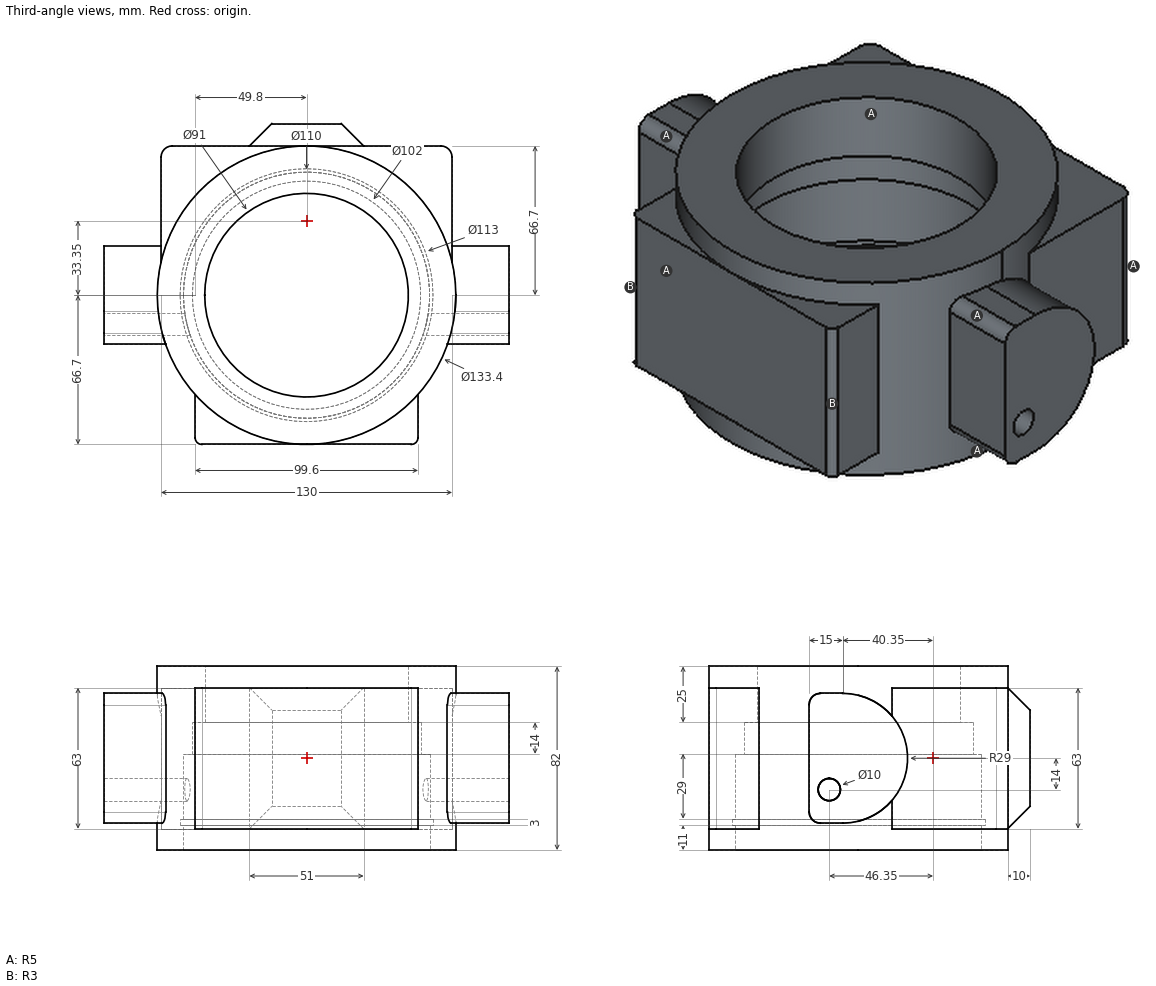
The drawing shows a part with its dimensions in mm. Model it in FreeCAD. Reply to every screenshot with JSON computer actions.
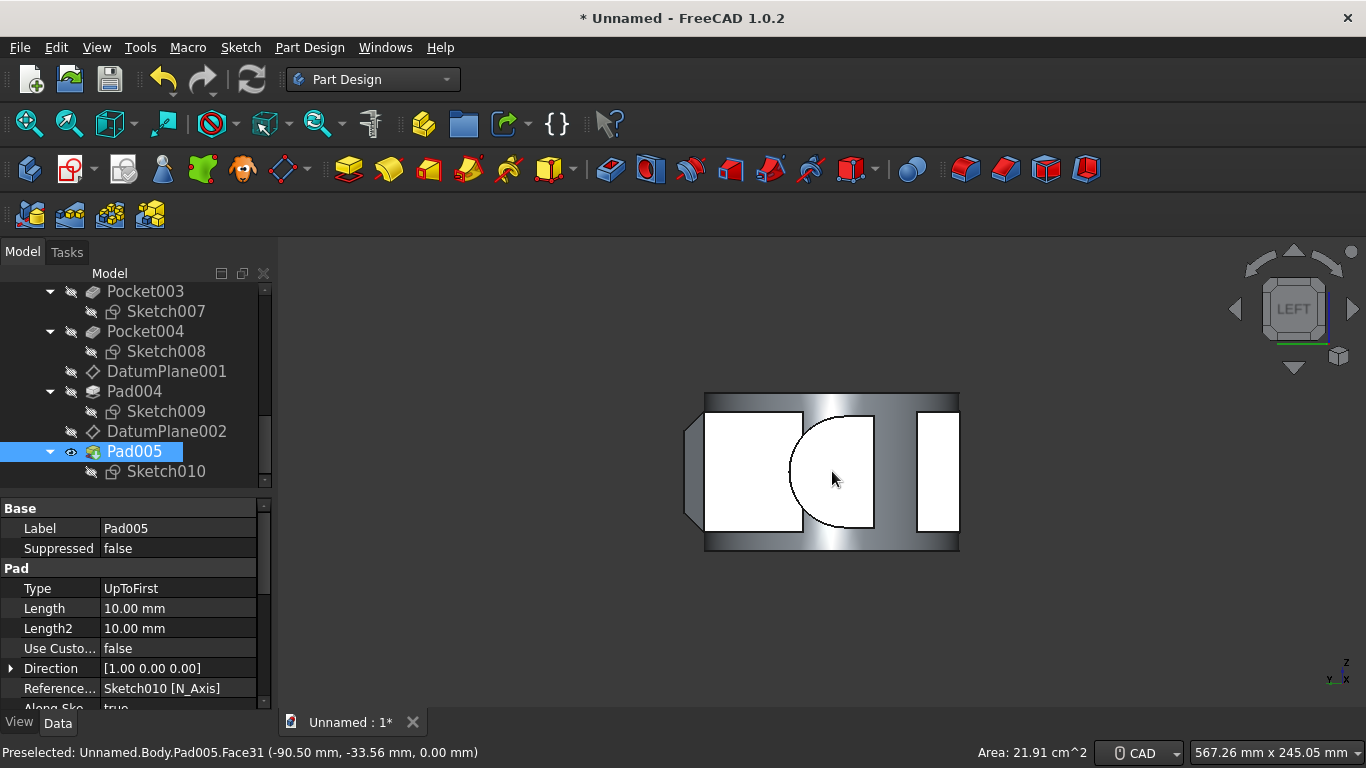
{"action": "left_click", "coordinate": [70, 170]}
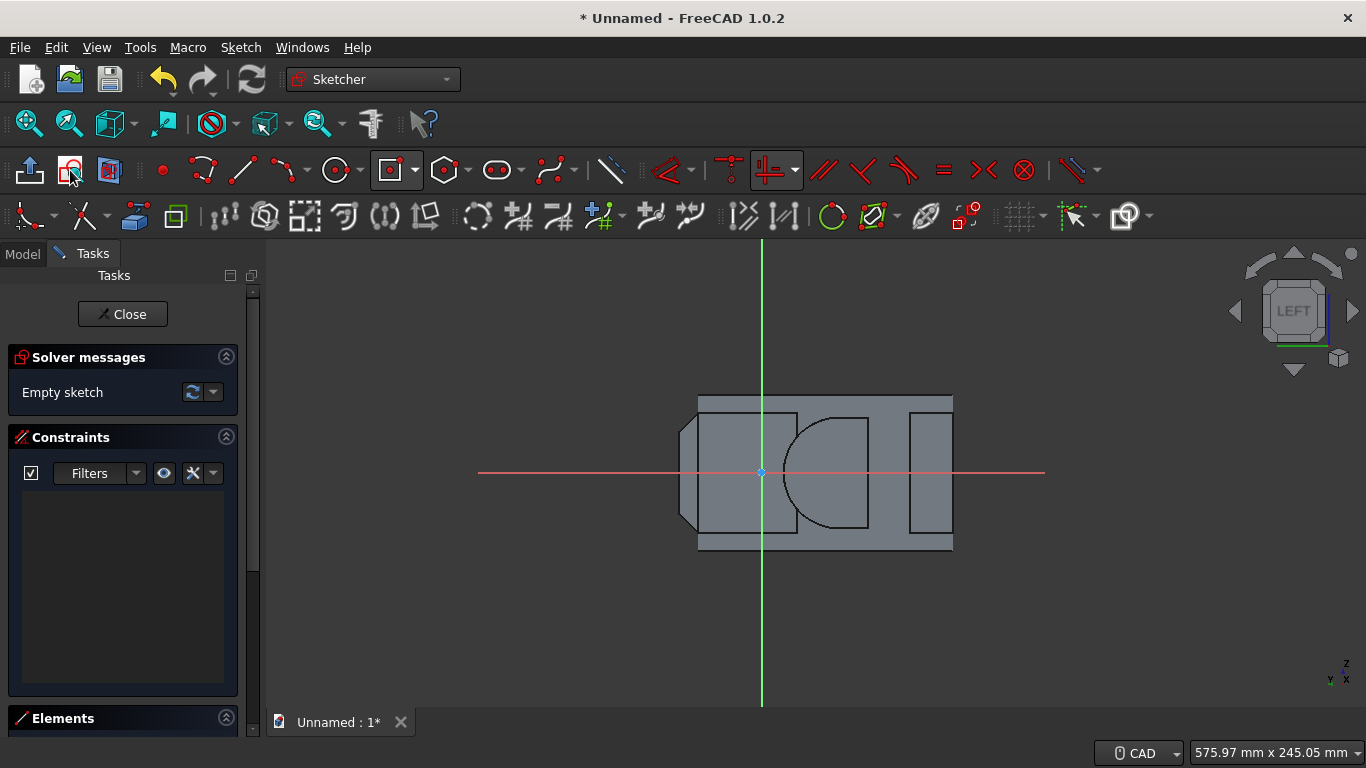
{"action": "scroll", "coordinate": [857, 501], "scroll_direction": "up", "scroll_amount": 14}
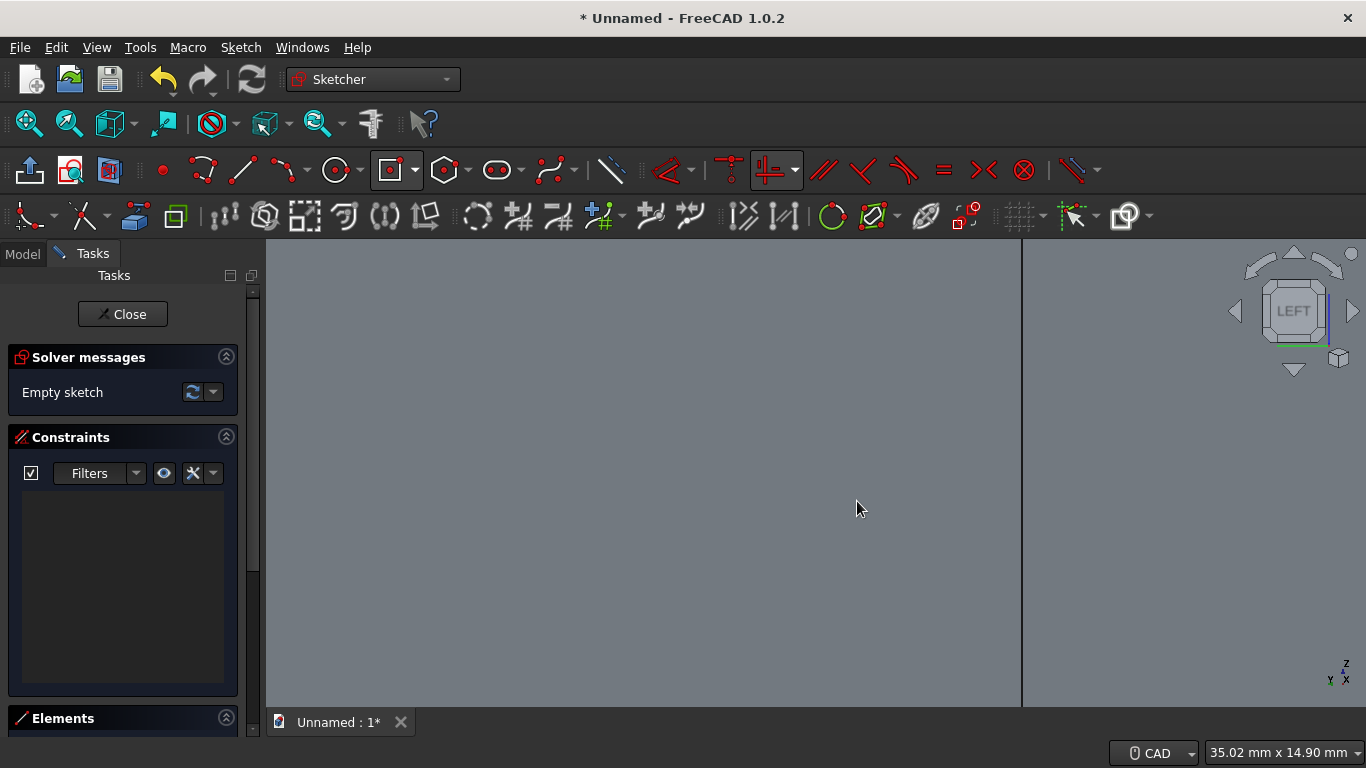
{"action": "left_click", "coordinate": [336, 170]}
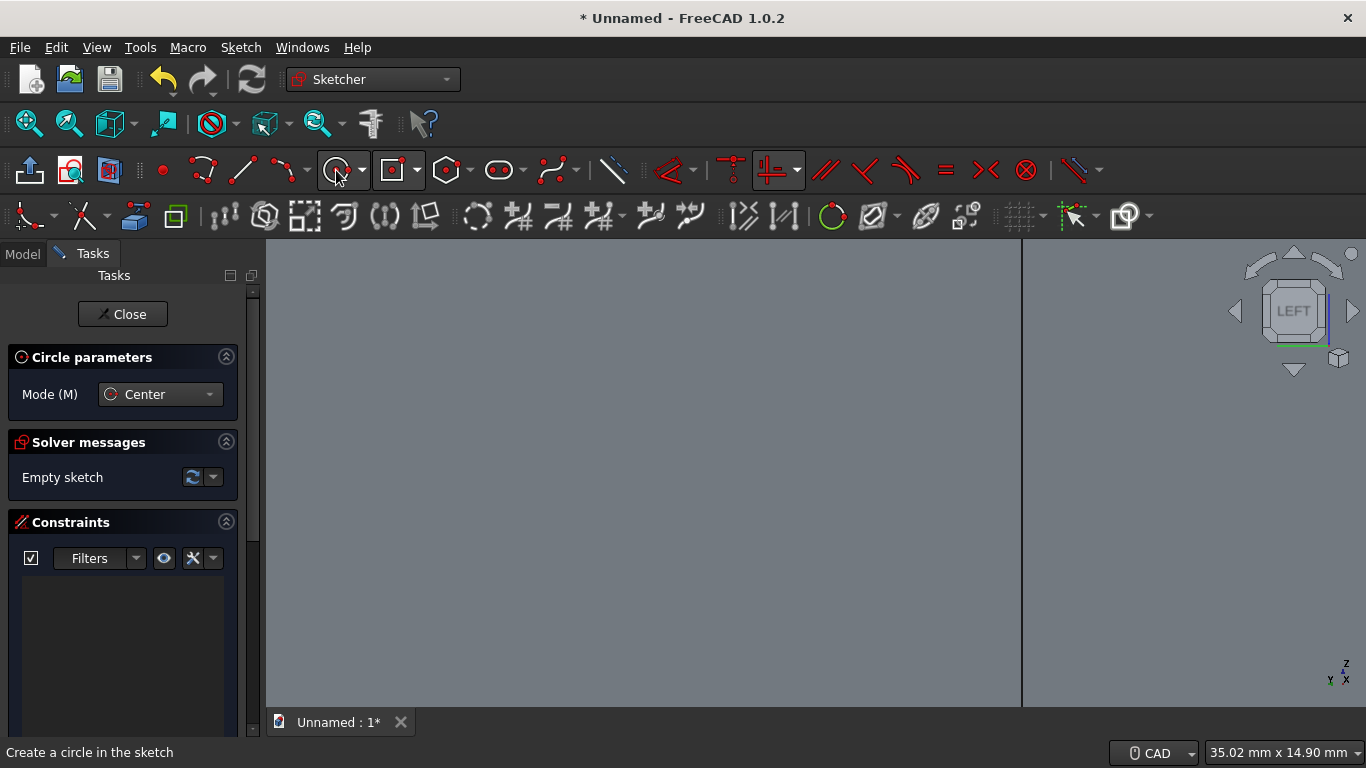
{"action": "left_click", "coordinate": [740, 472]}
{"action": "left_click", "coordinate": [851, 361]}
{"action": "key", "text": "Escape"}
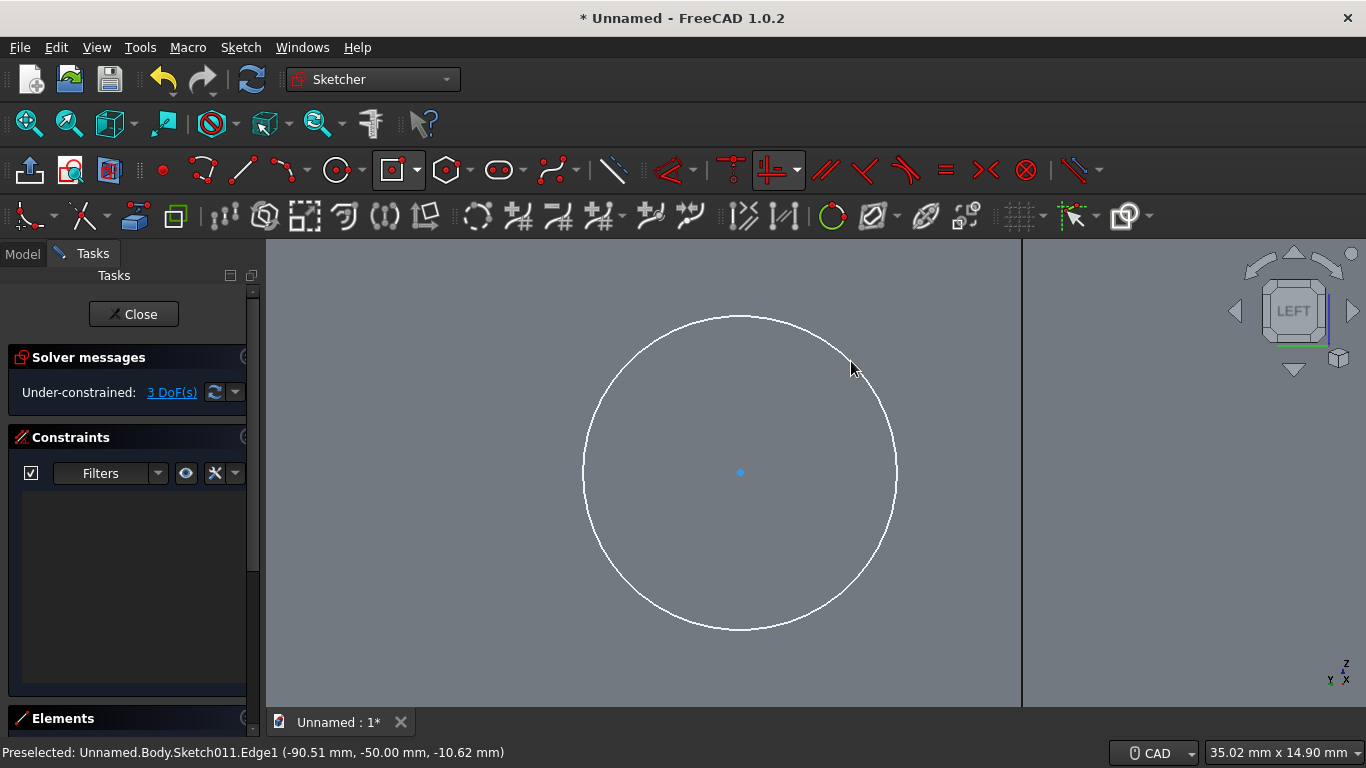
{"action": "key", "text": "d"}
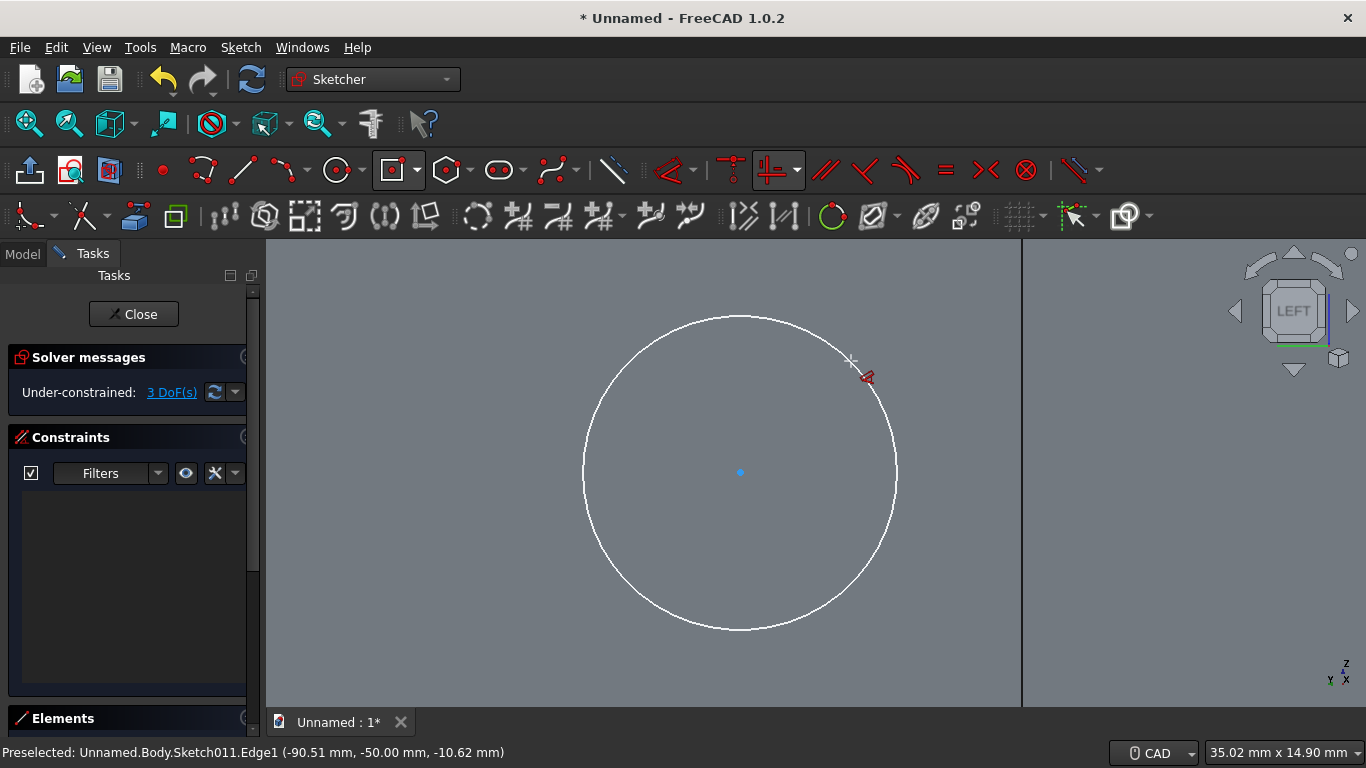
{"action": "left_click", "coordinate": [851, 362]}
{"action": "left_click", "coordinate": [874, 339]}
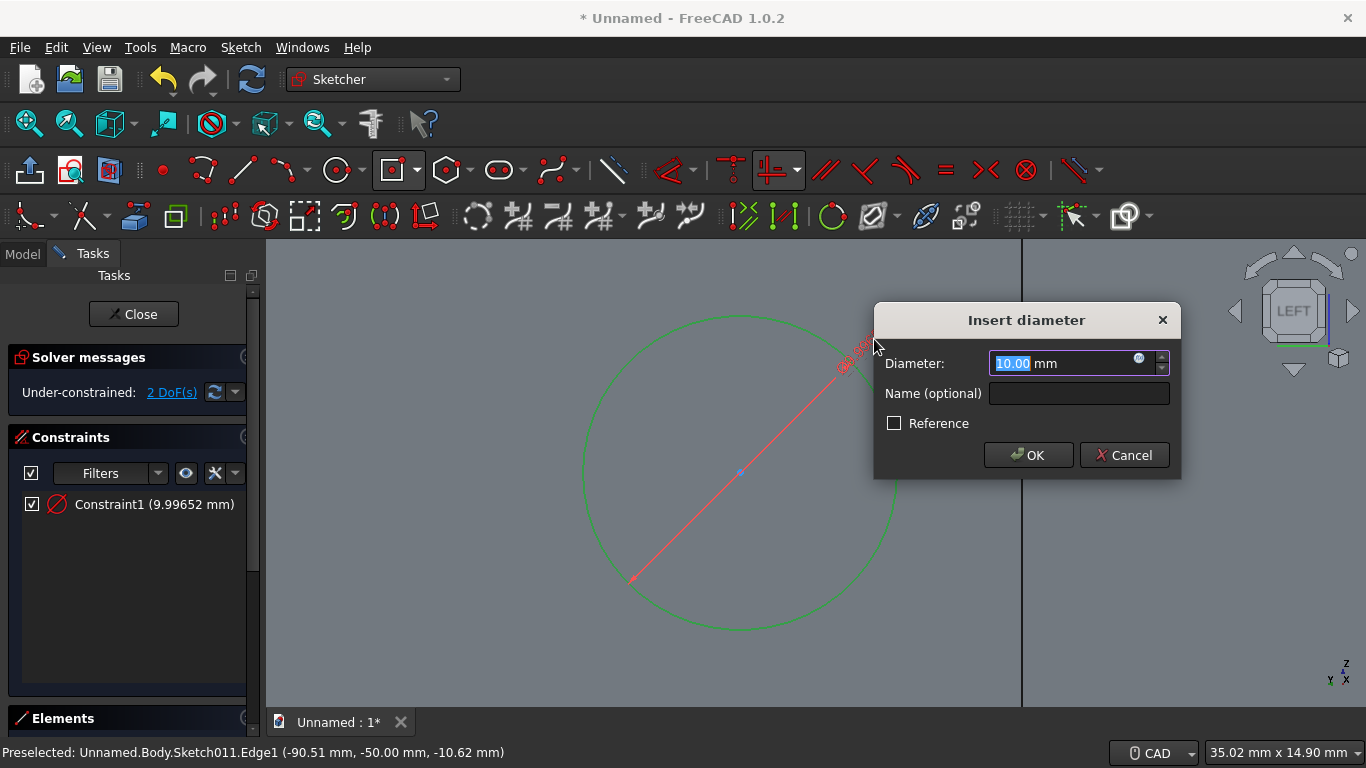
{"action": "type", "text": "10"}
{"action": "key", "text": "Return"}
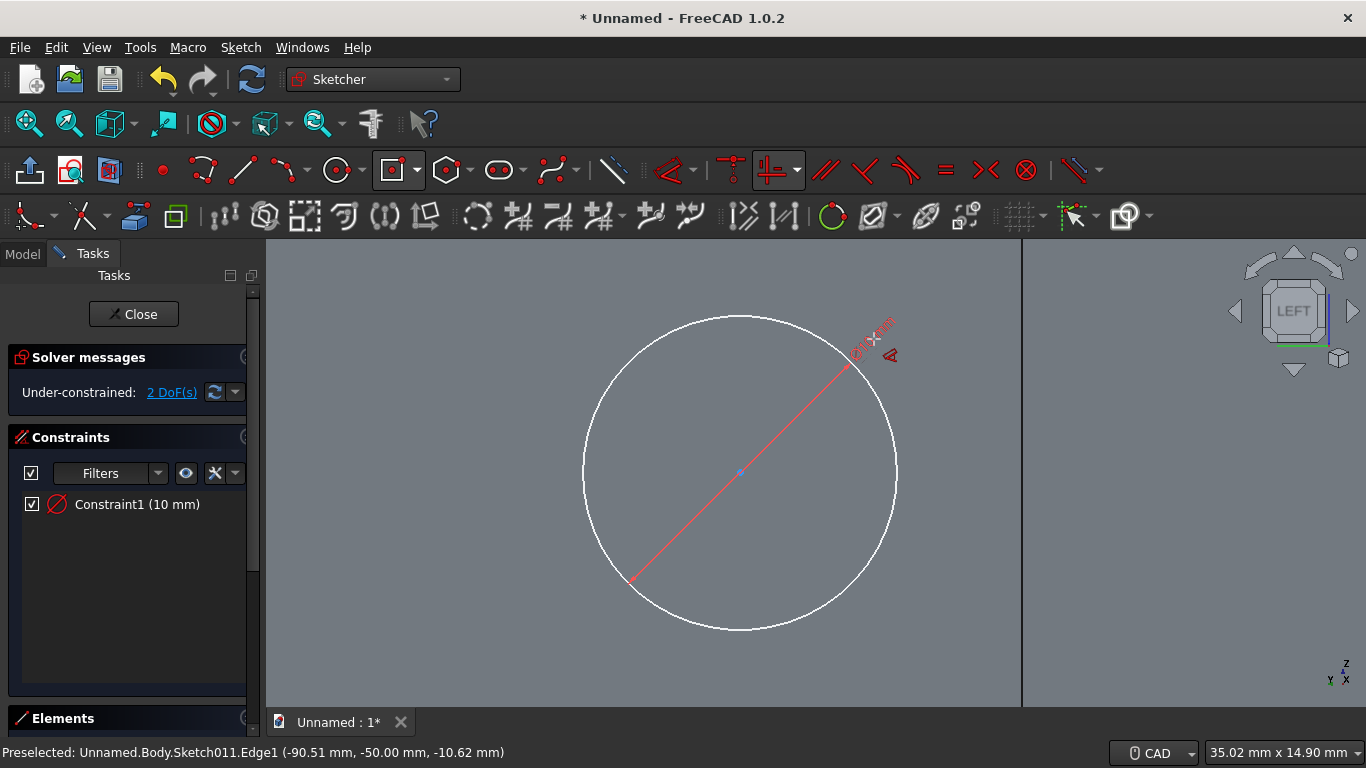
{"action": "left_click", "coordinate": [740, 473]}
{"action": "left_click", "coordinate": [774, 370]}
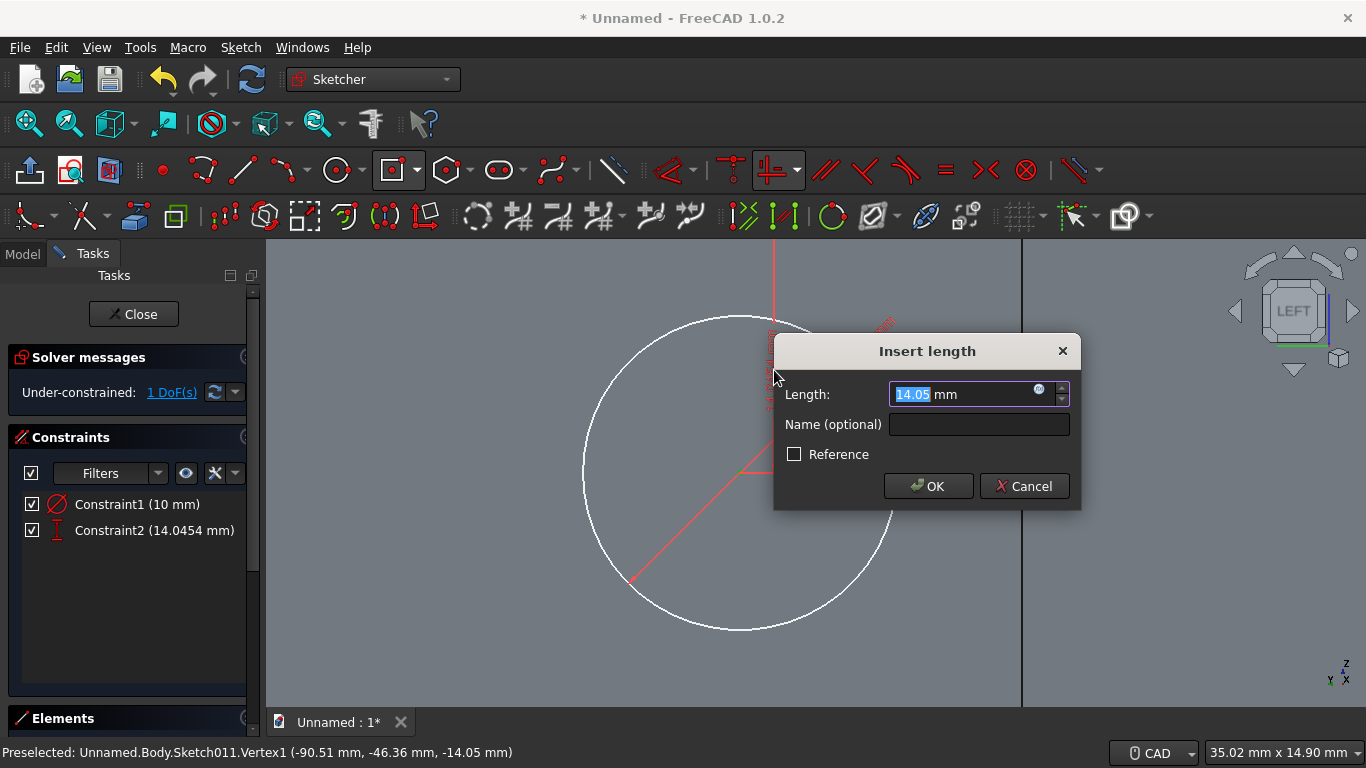
{"action": "type", "text": "14"}
{"action": "key", "text": "Return"}